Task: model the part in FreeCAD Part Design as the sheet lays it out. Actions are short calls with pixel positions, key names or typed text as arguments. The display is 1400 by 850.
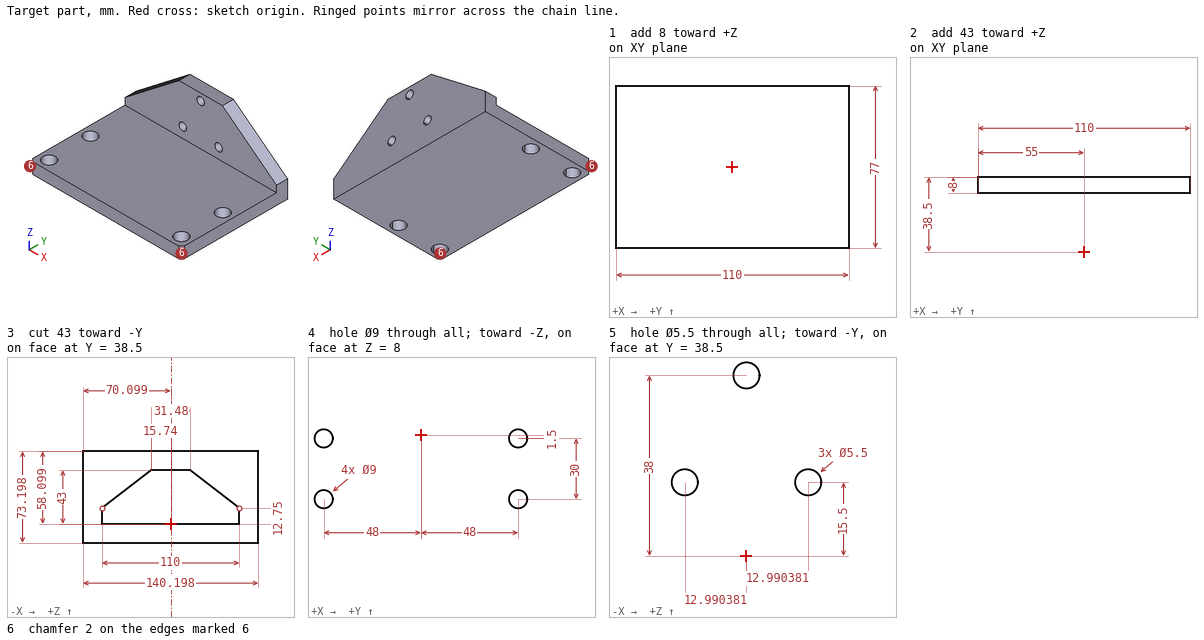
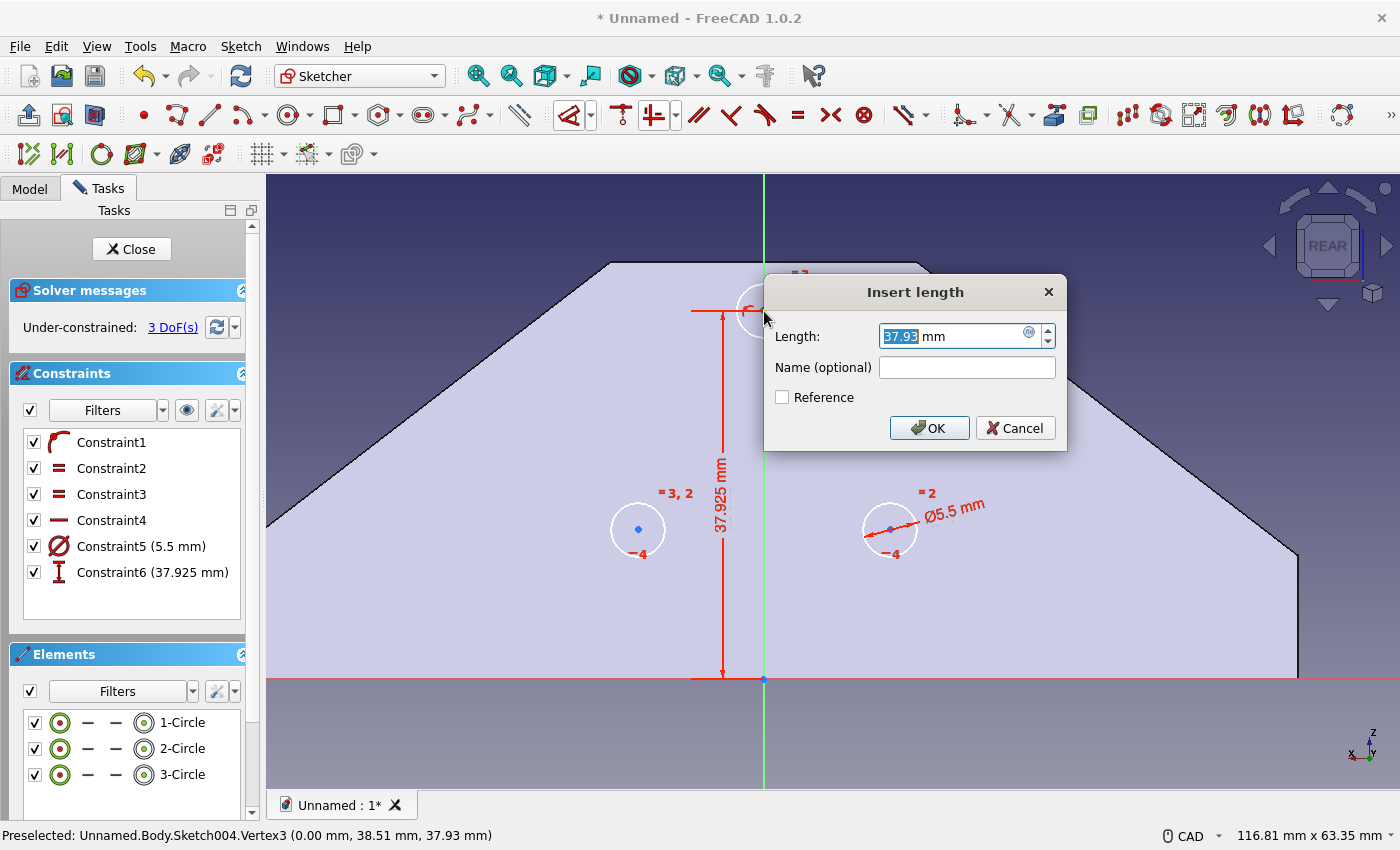
text(38)
key(Return)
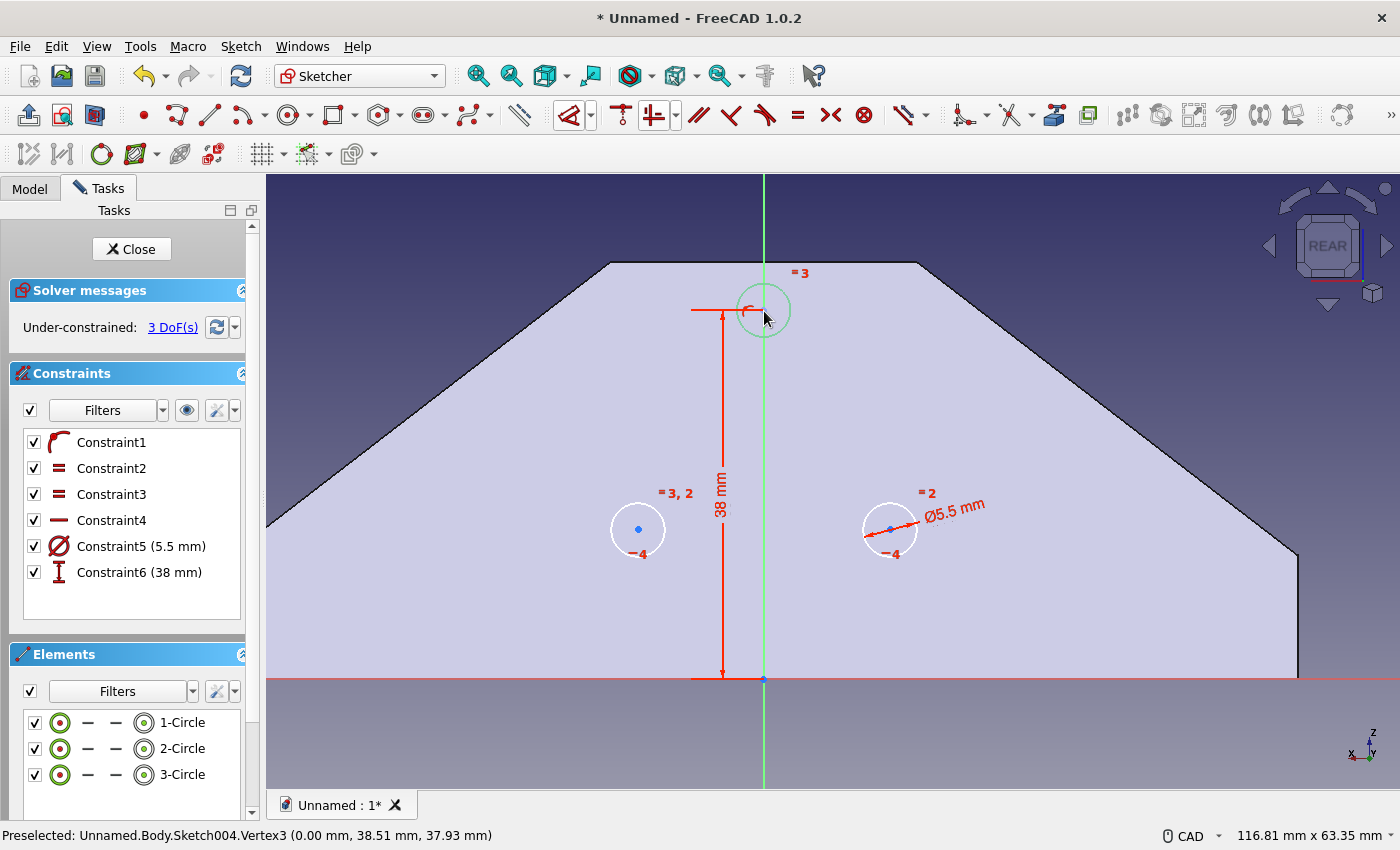
click(890, 530)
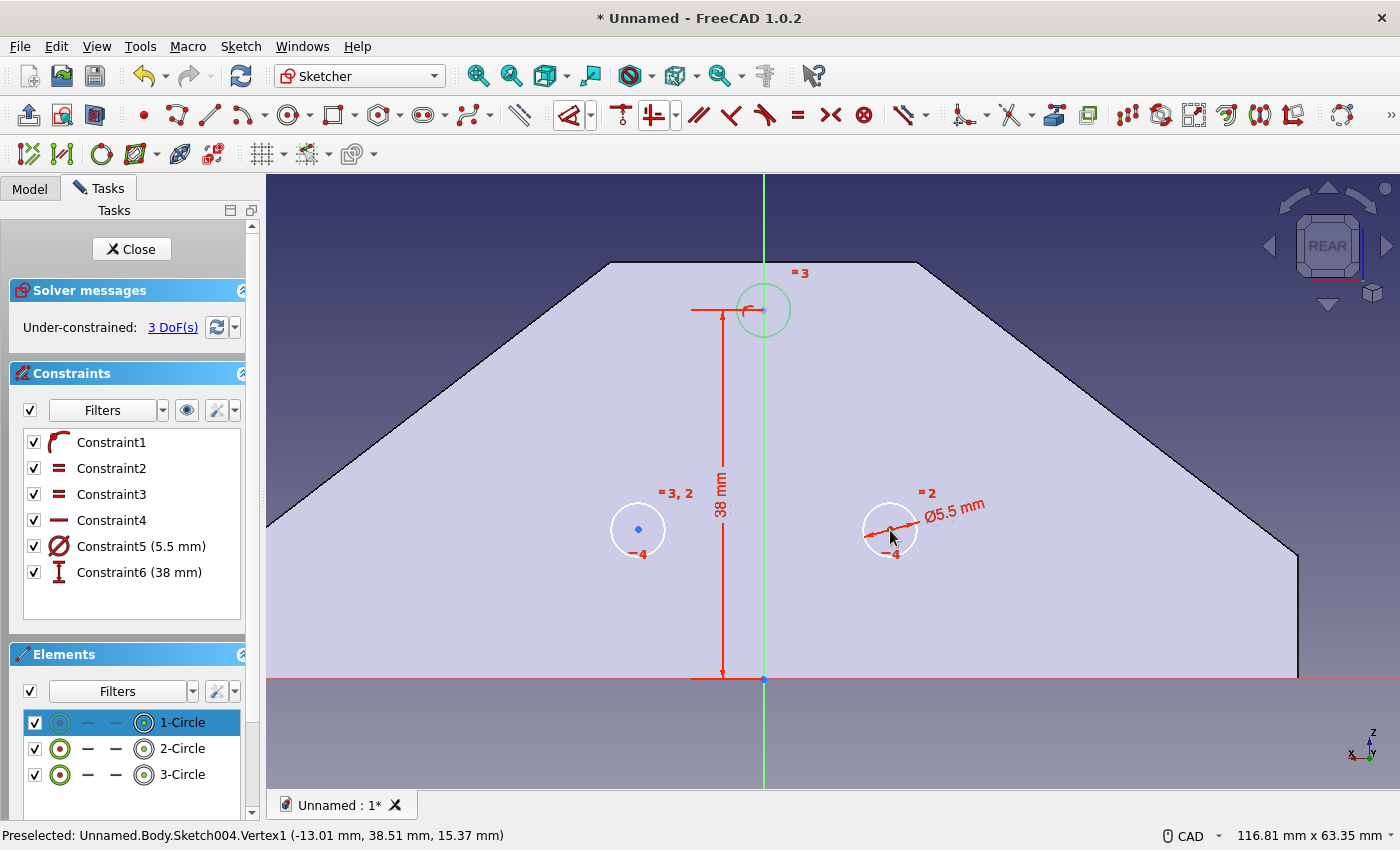
key(i)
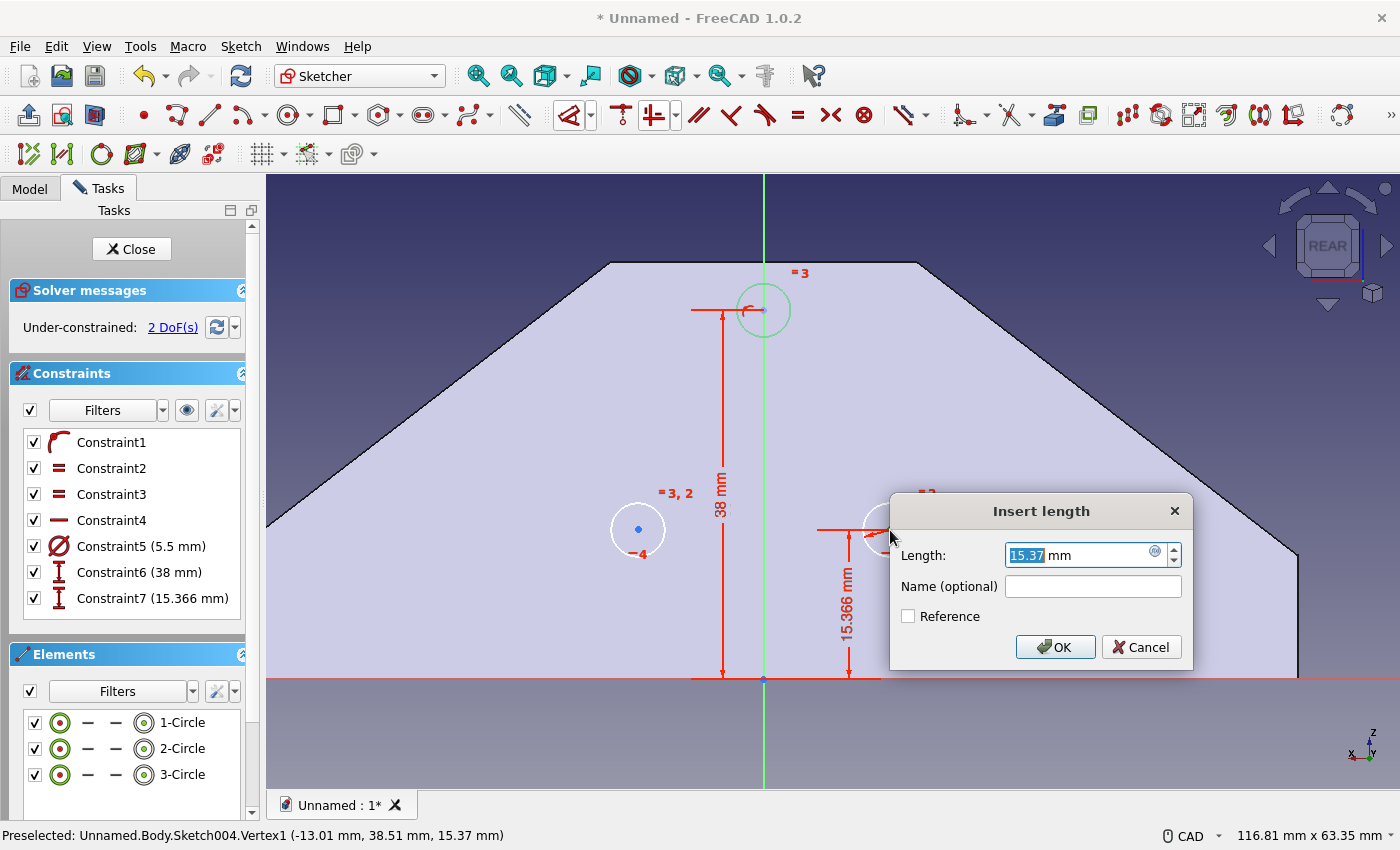
text(15.5)
key(Return)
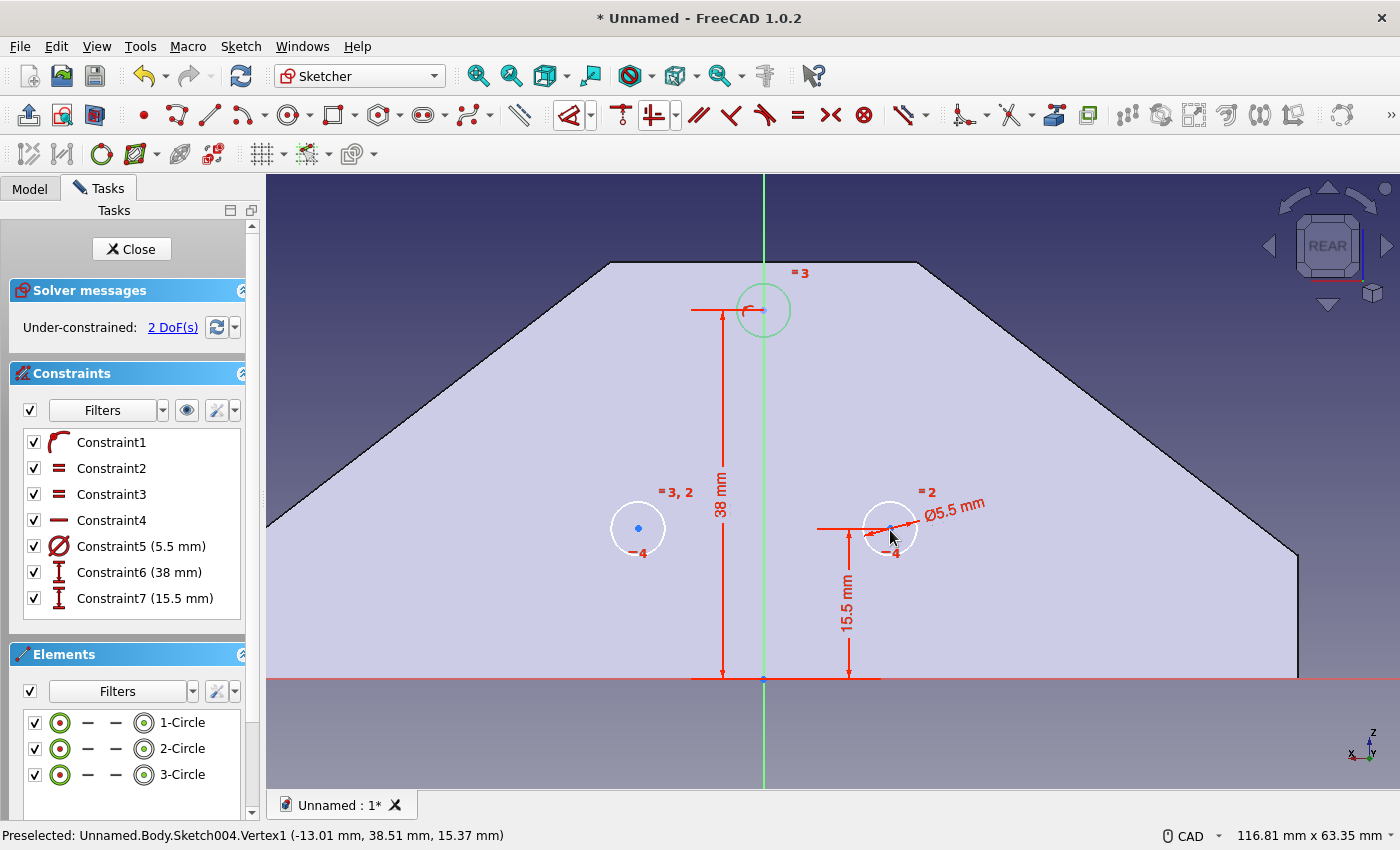
click(890, 529)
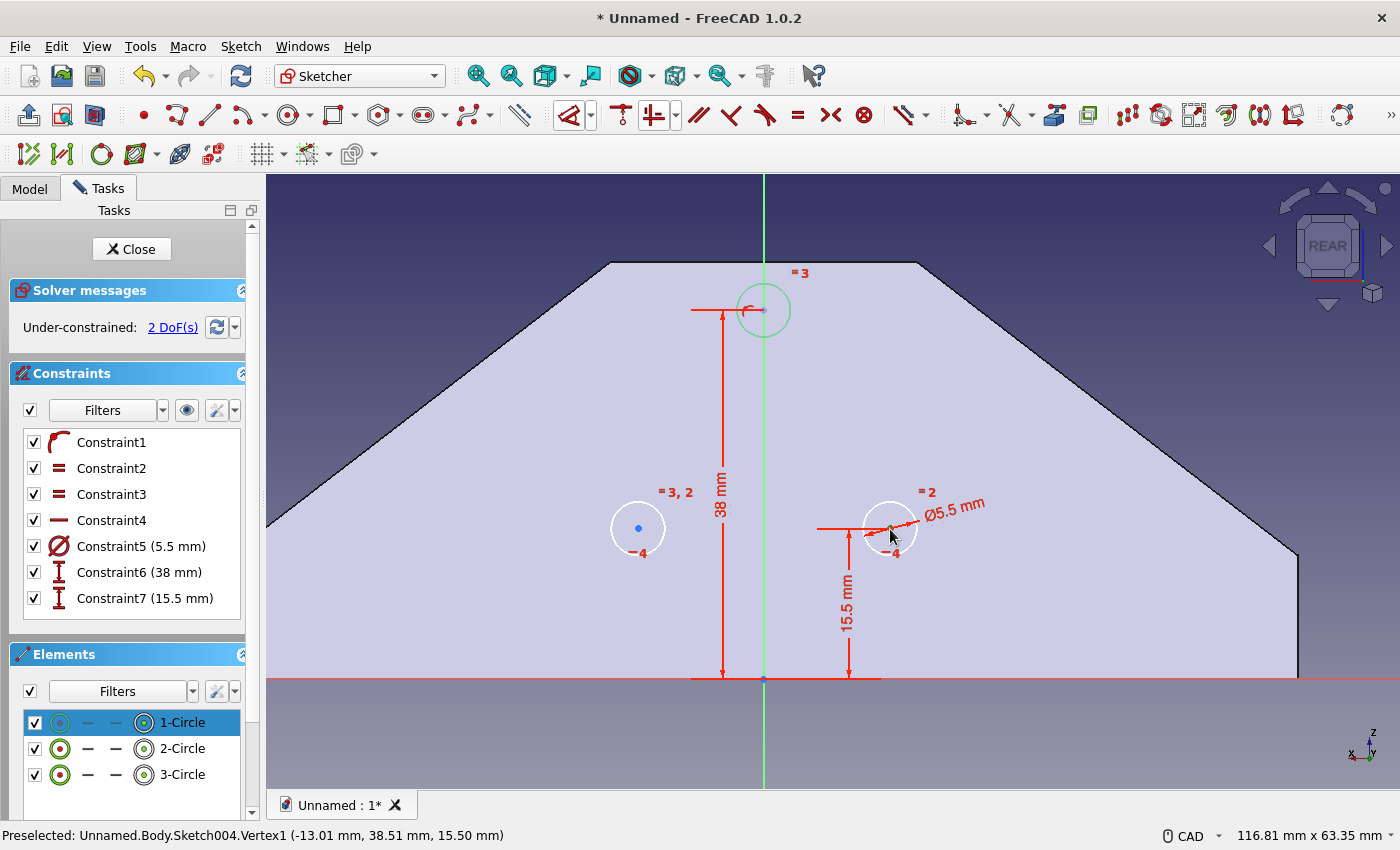
key(l)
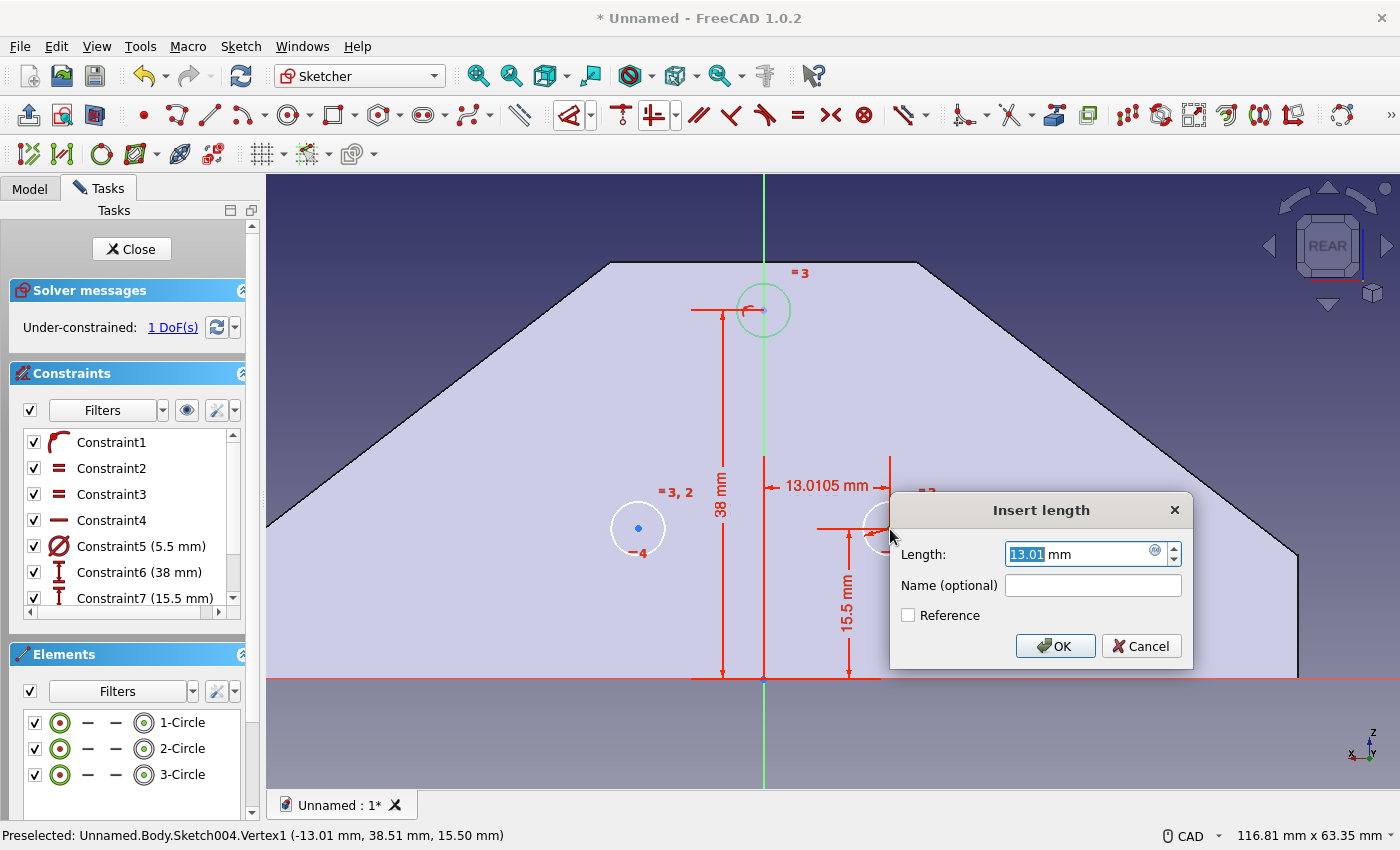
text(12.990381)
key(Return)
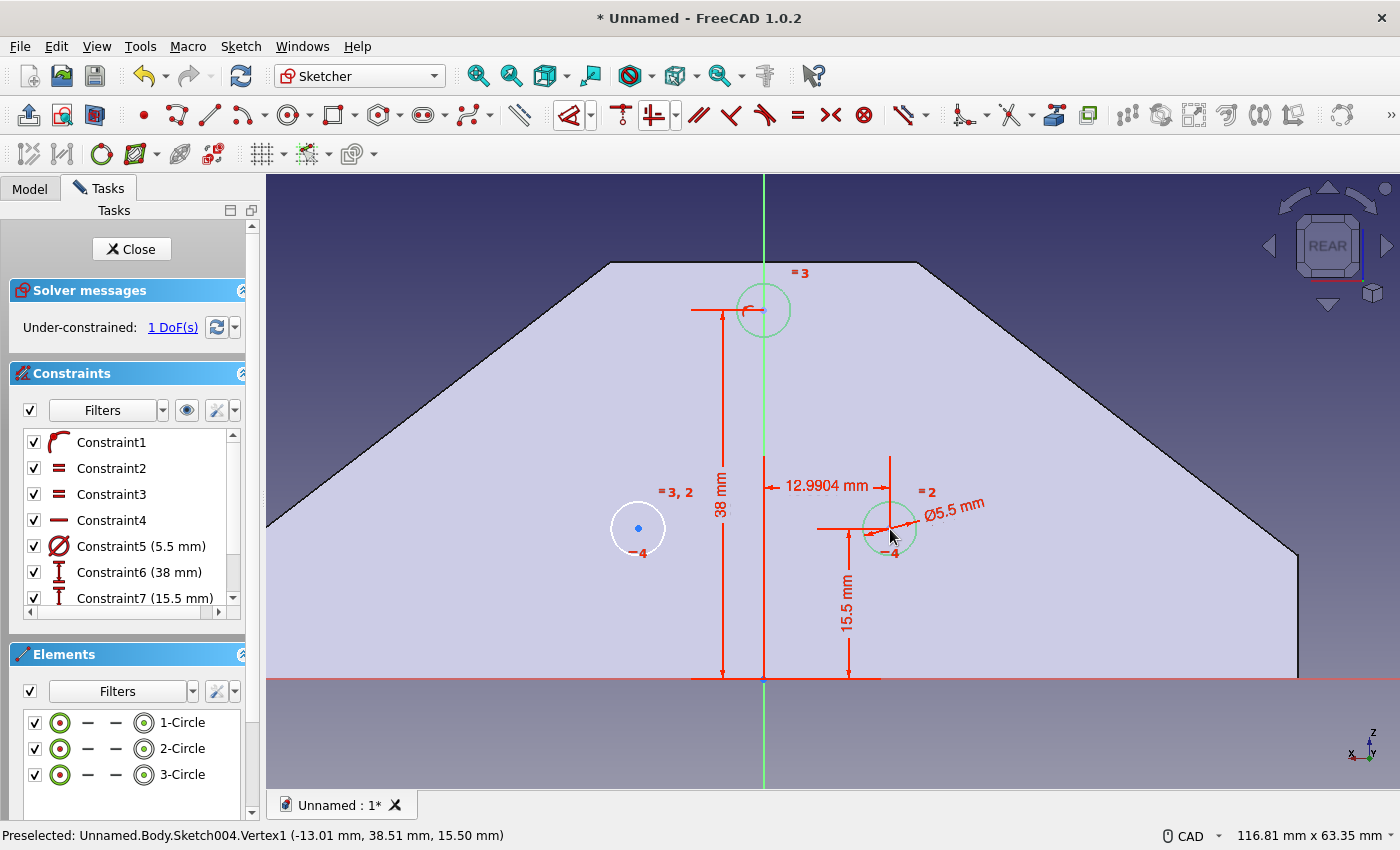
click(638, 529)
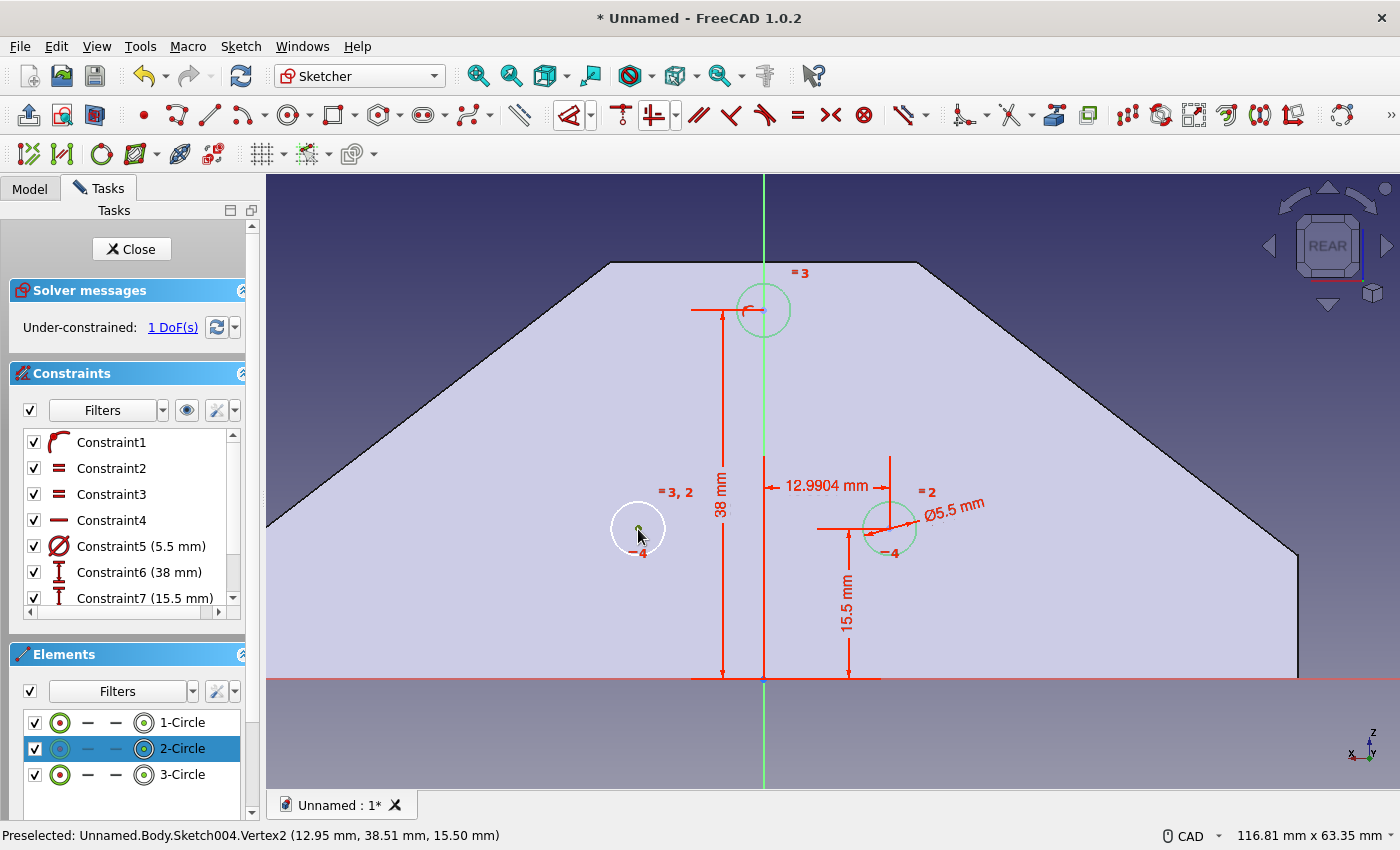
key(l)